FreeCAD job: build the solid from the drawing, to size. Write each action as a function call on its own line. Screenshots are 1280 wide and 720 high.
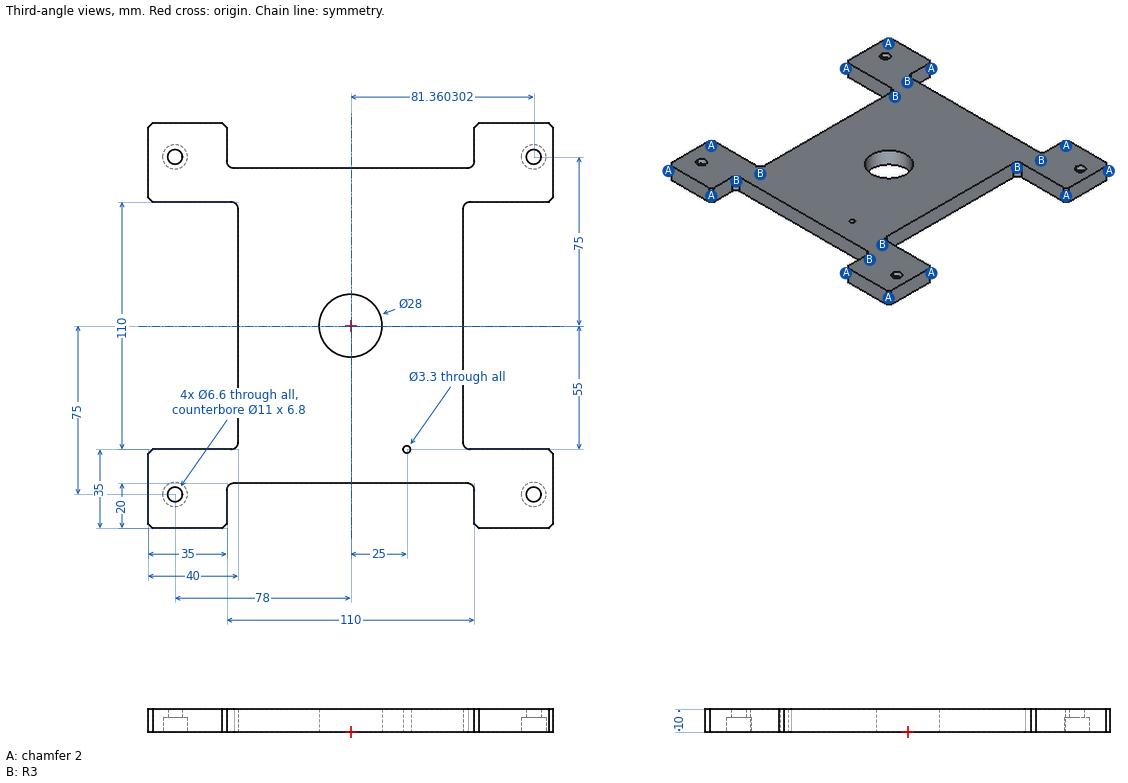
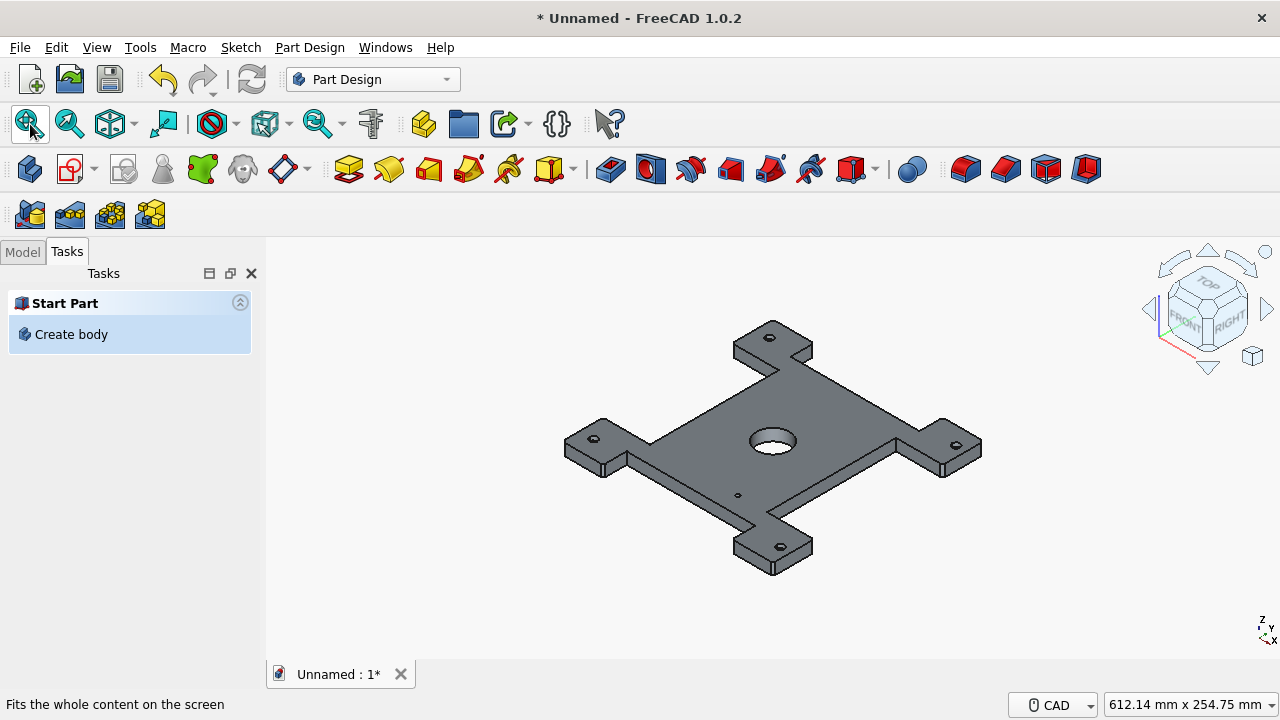
key(2)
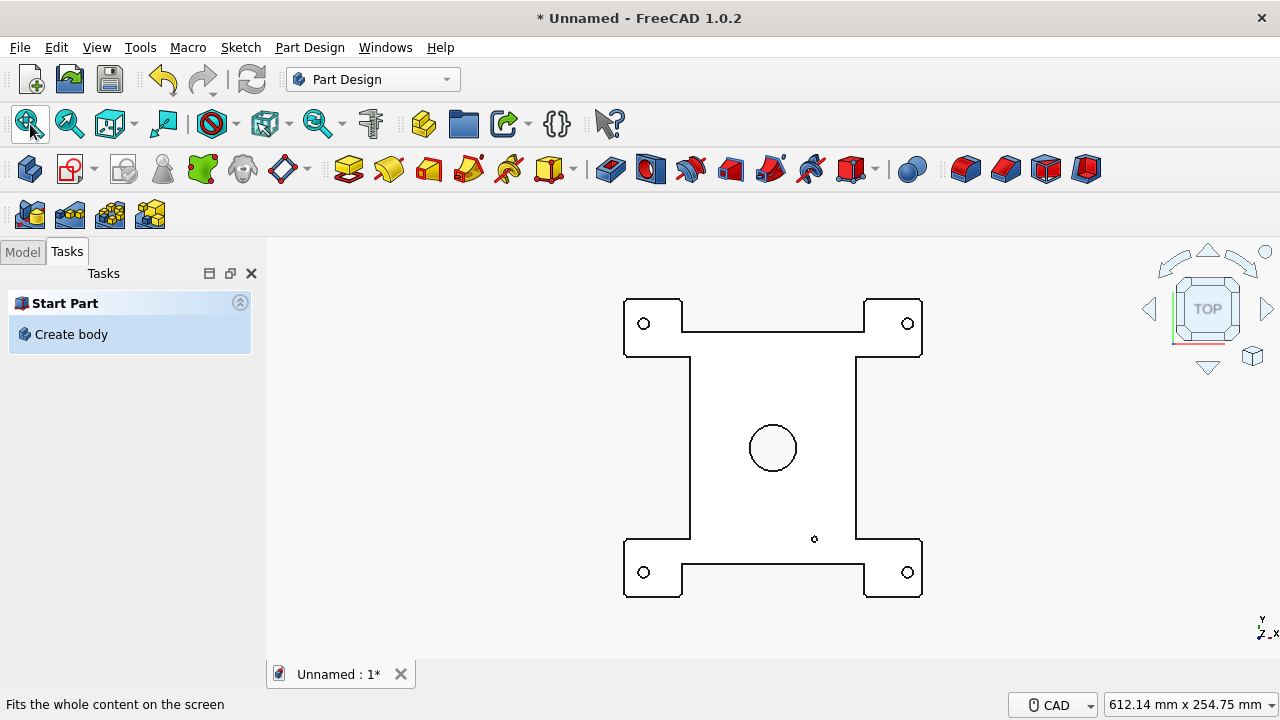
scroll(682, 331, up, 5)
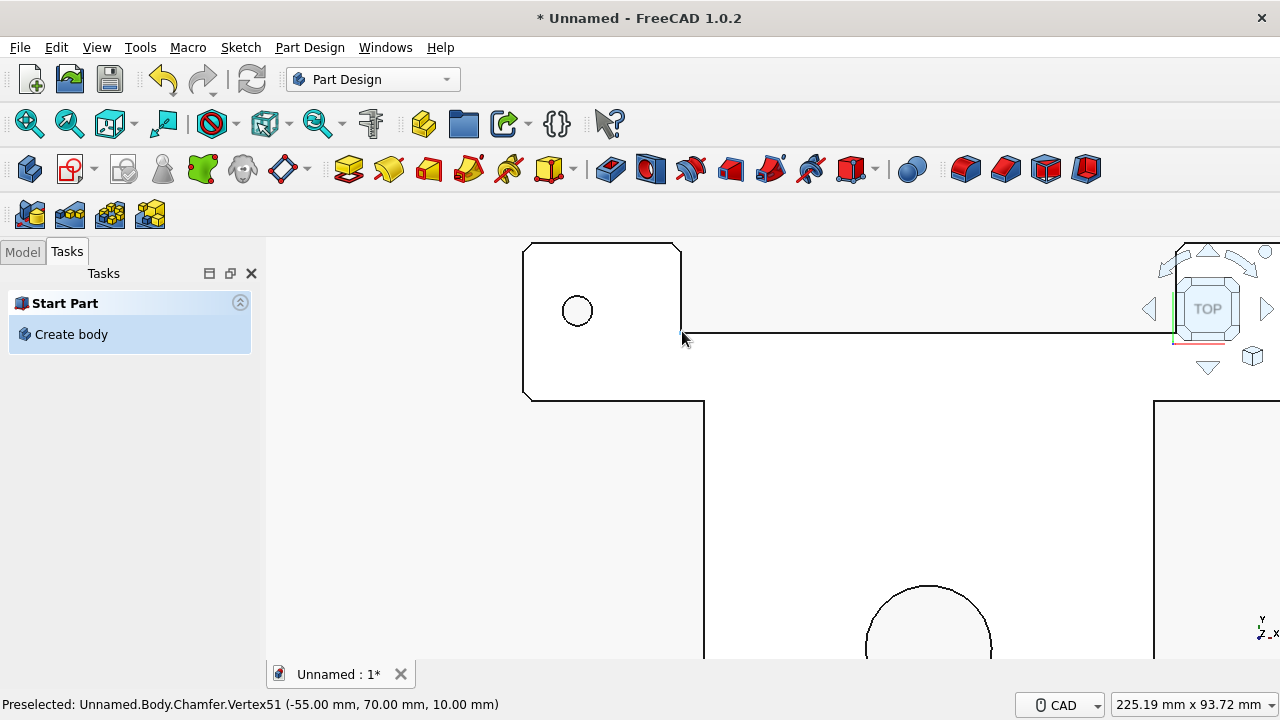
click(30, 124)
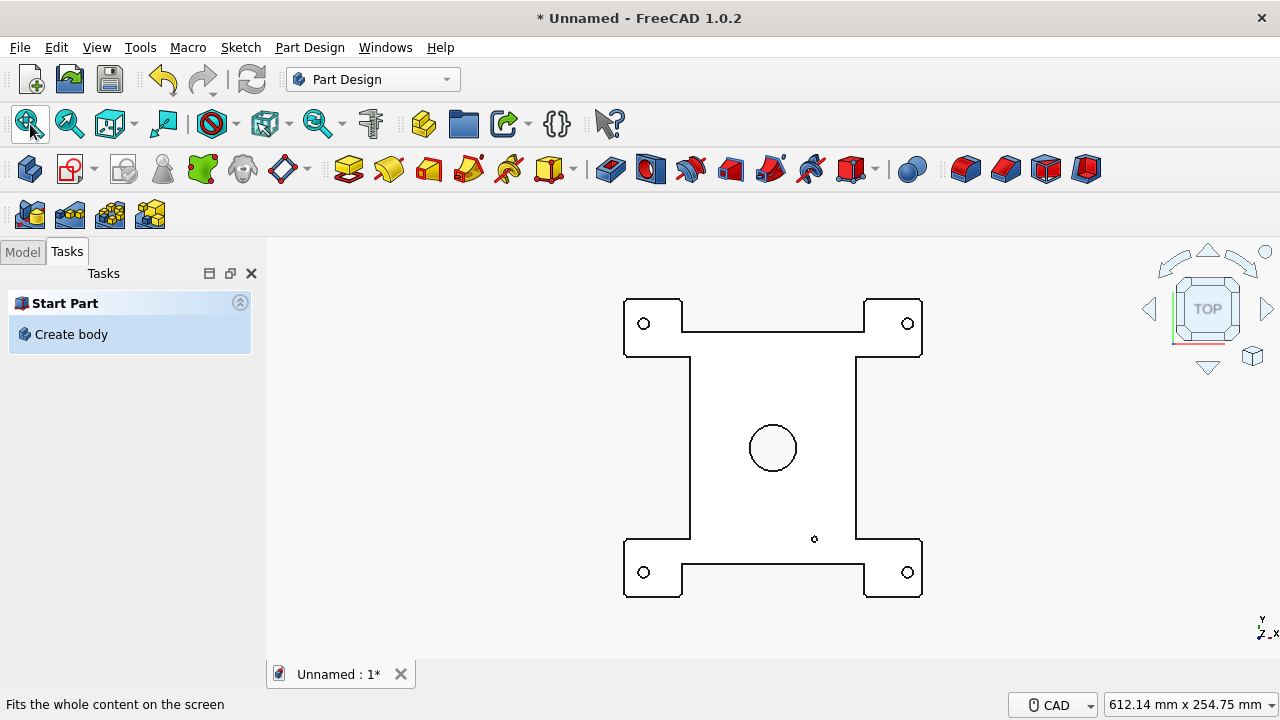
key(1)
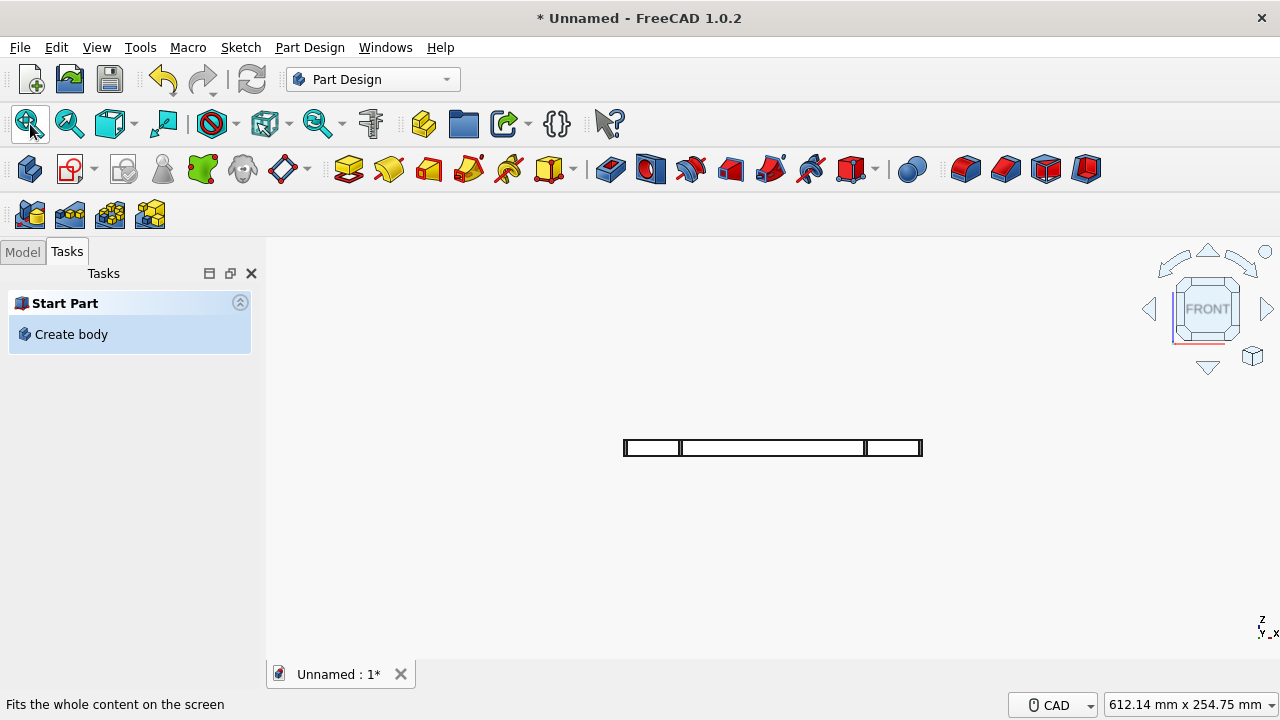
click(30, 124)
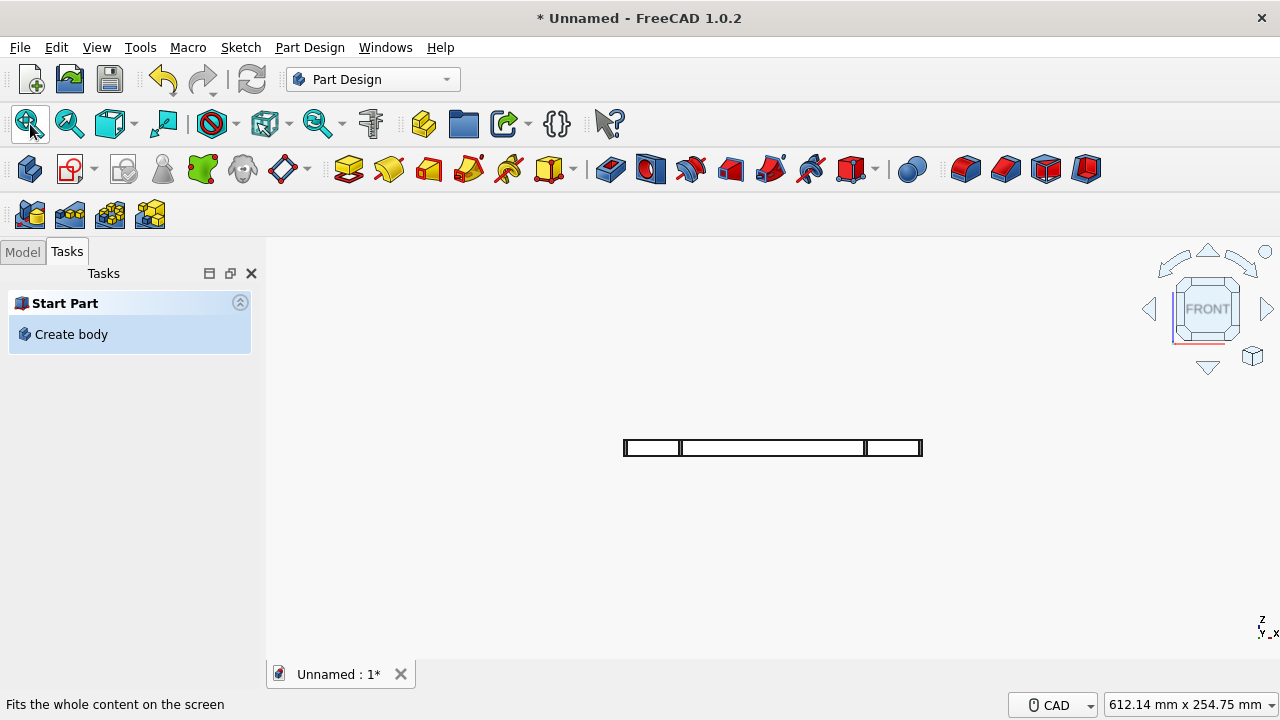
scroll(682, 447, up, 5)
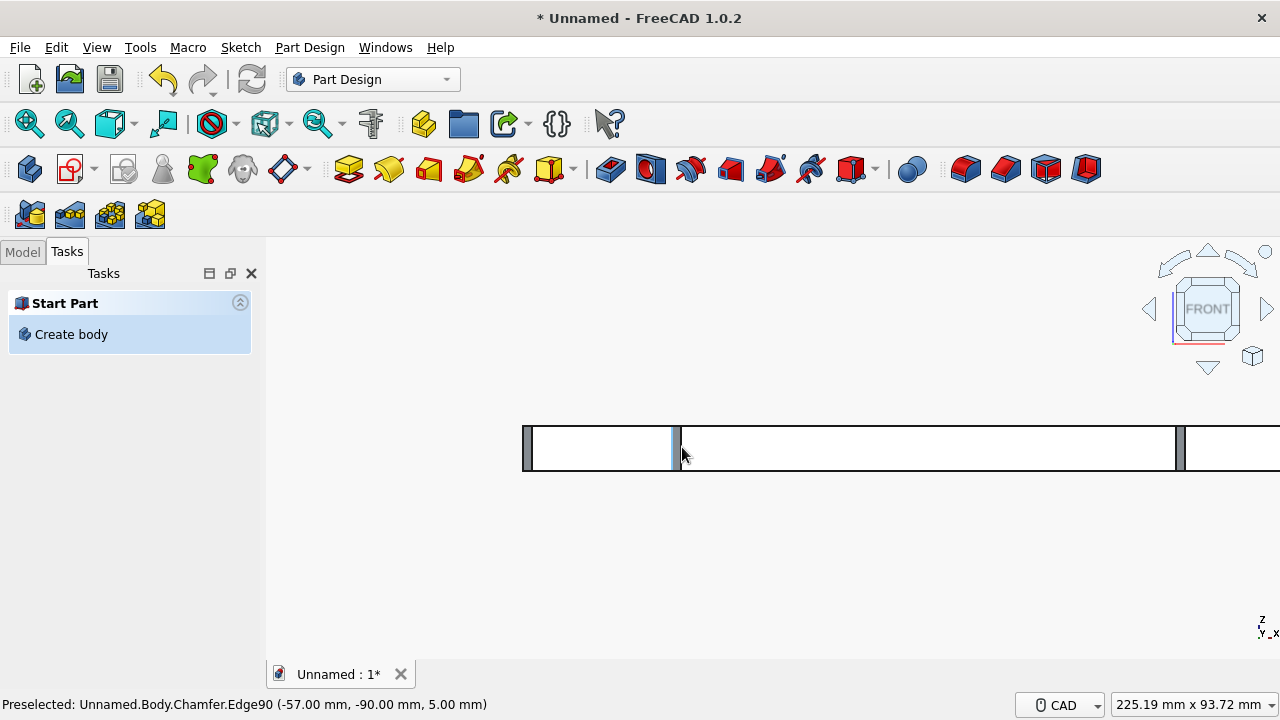
click(30, 124)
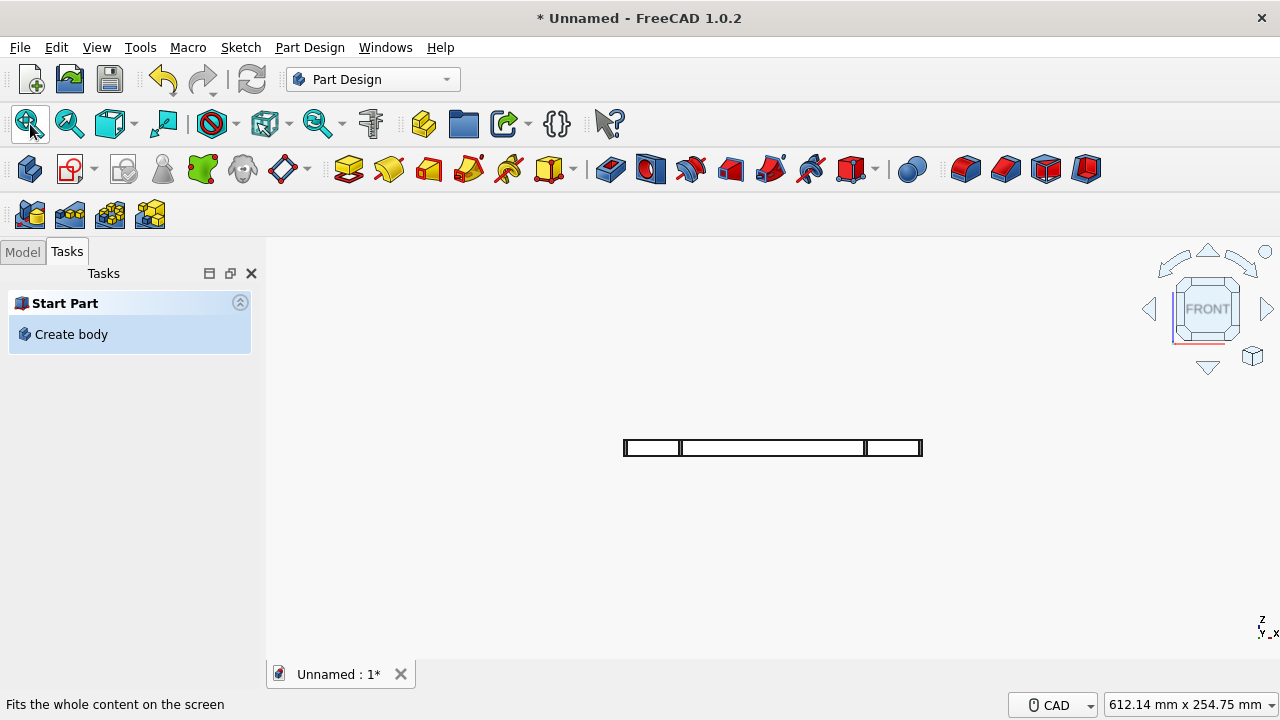
key(3)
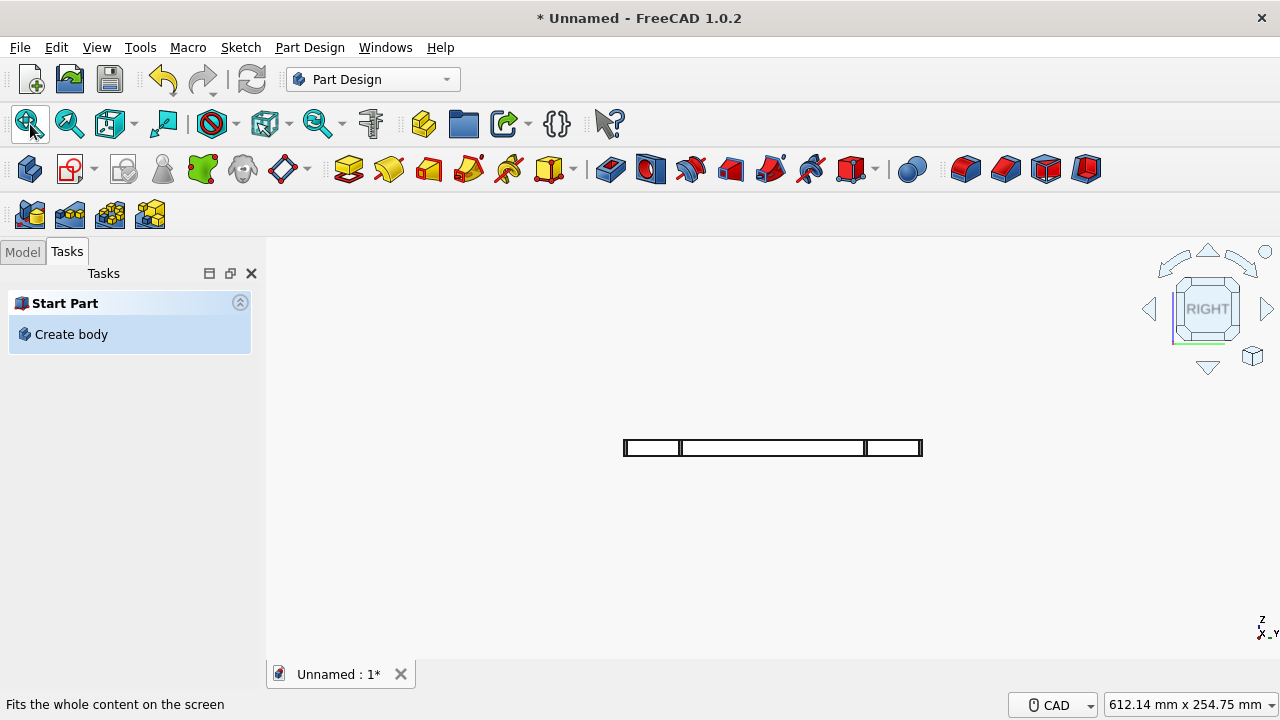
click(30, 124)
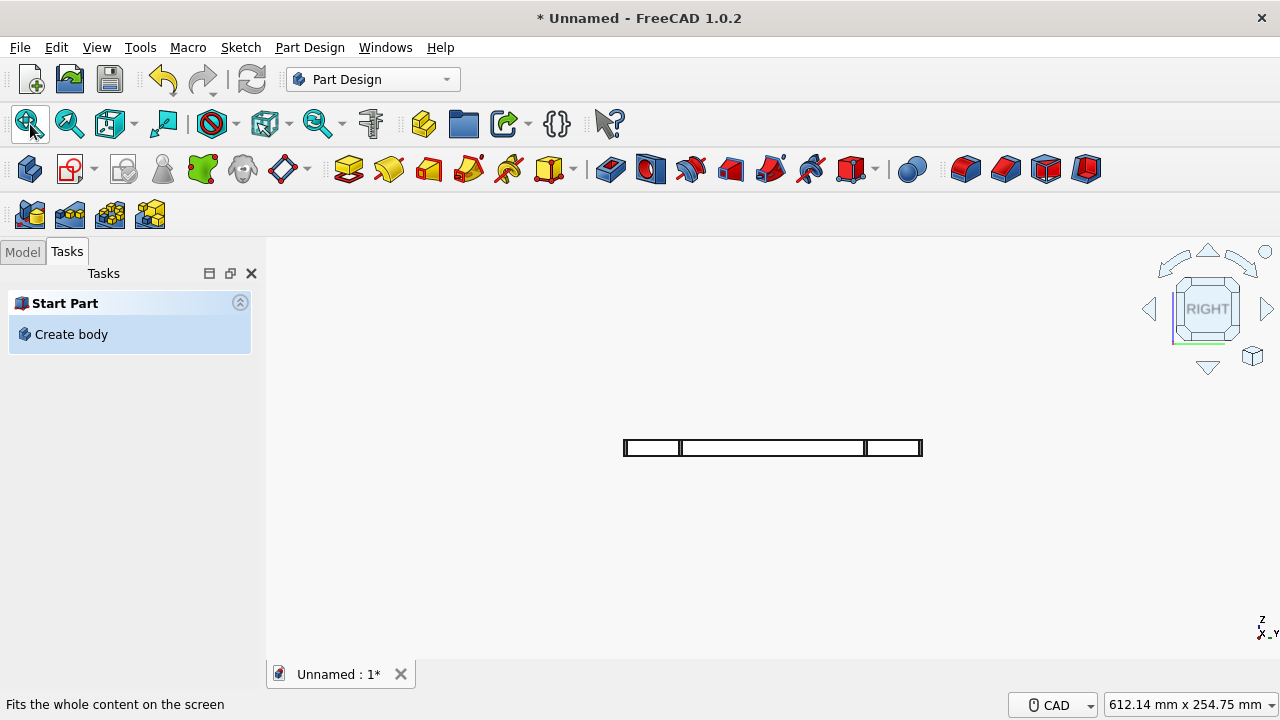
scroll(889, 447, up, 5)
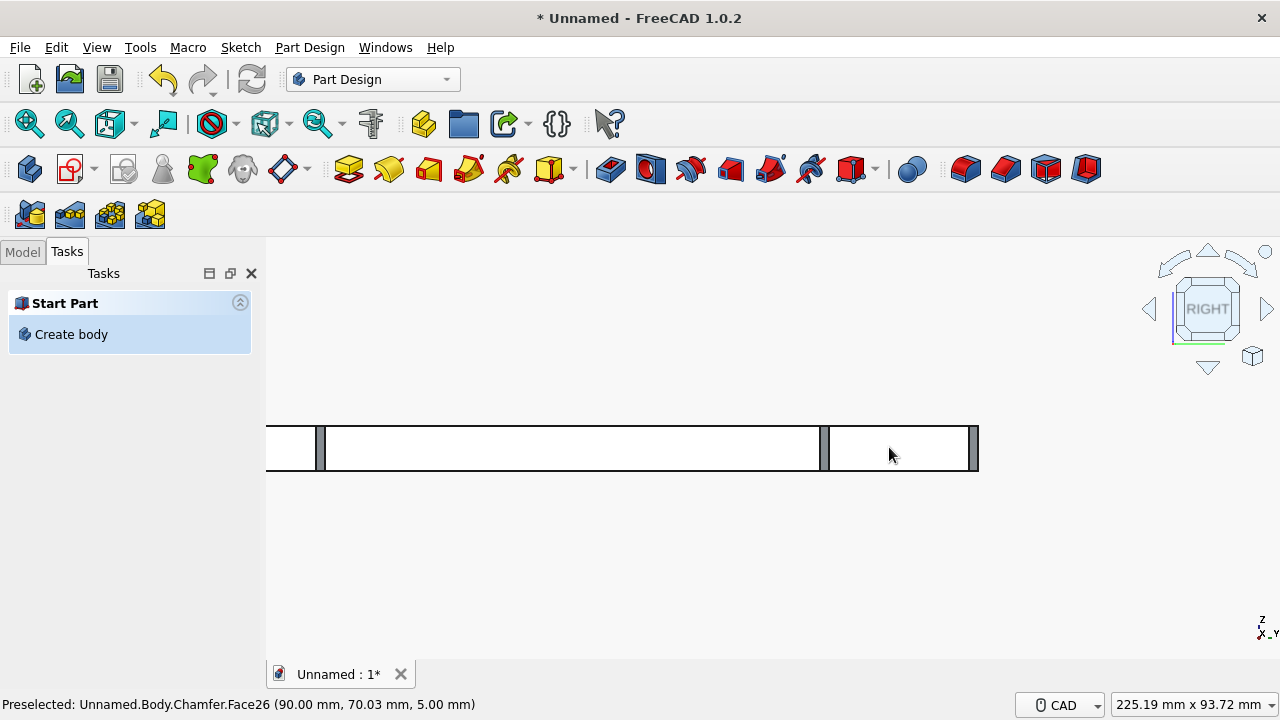
click(30, 124)